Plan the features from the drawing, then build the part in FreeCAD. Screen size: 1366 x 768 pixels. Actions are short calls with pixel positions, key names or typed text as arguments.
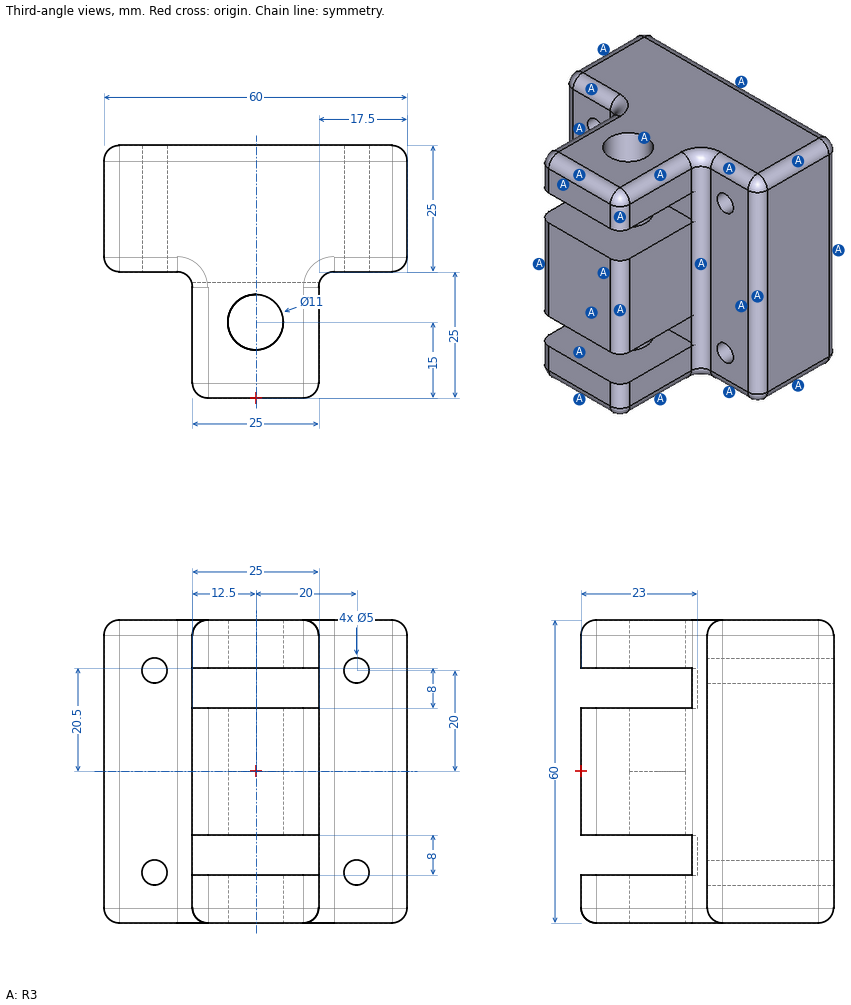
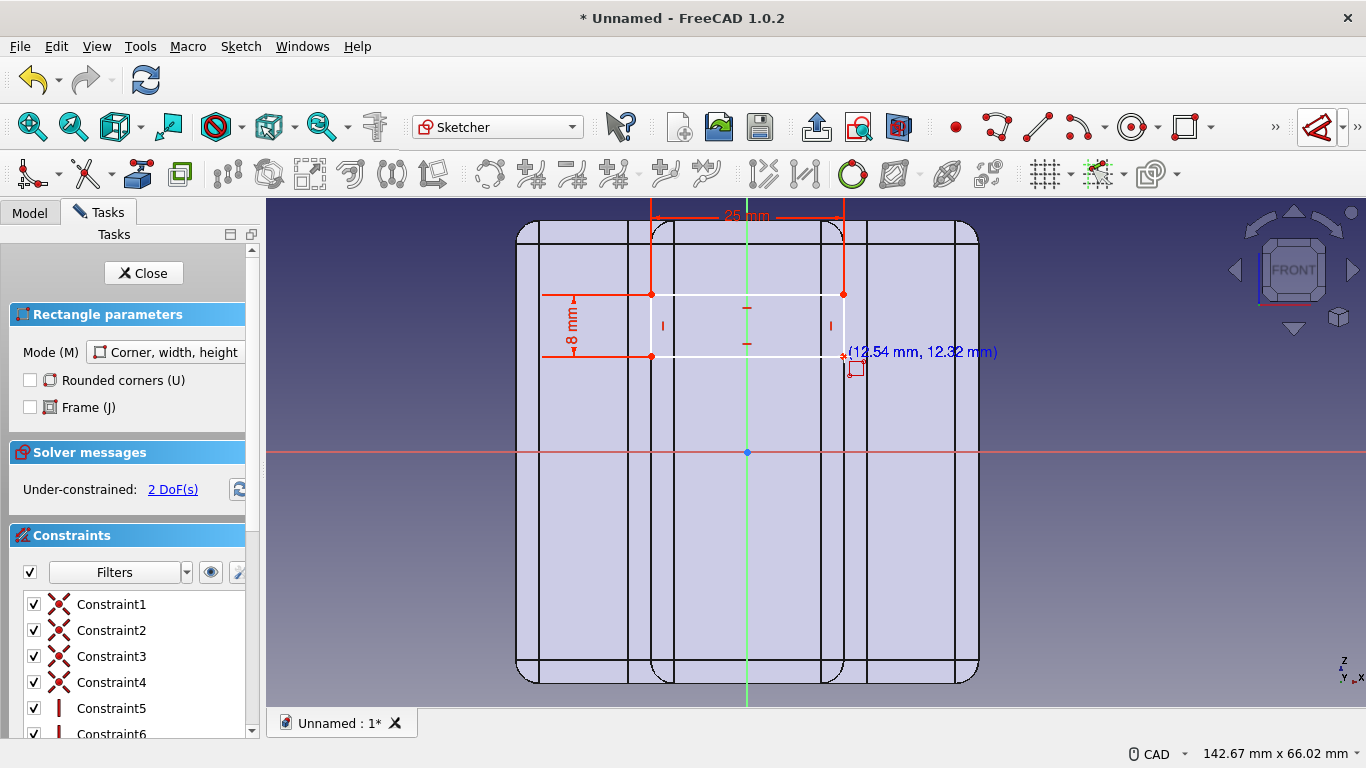
click(651, 548)
move(844, 610)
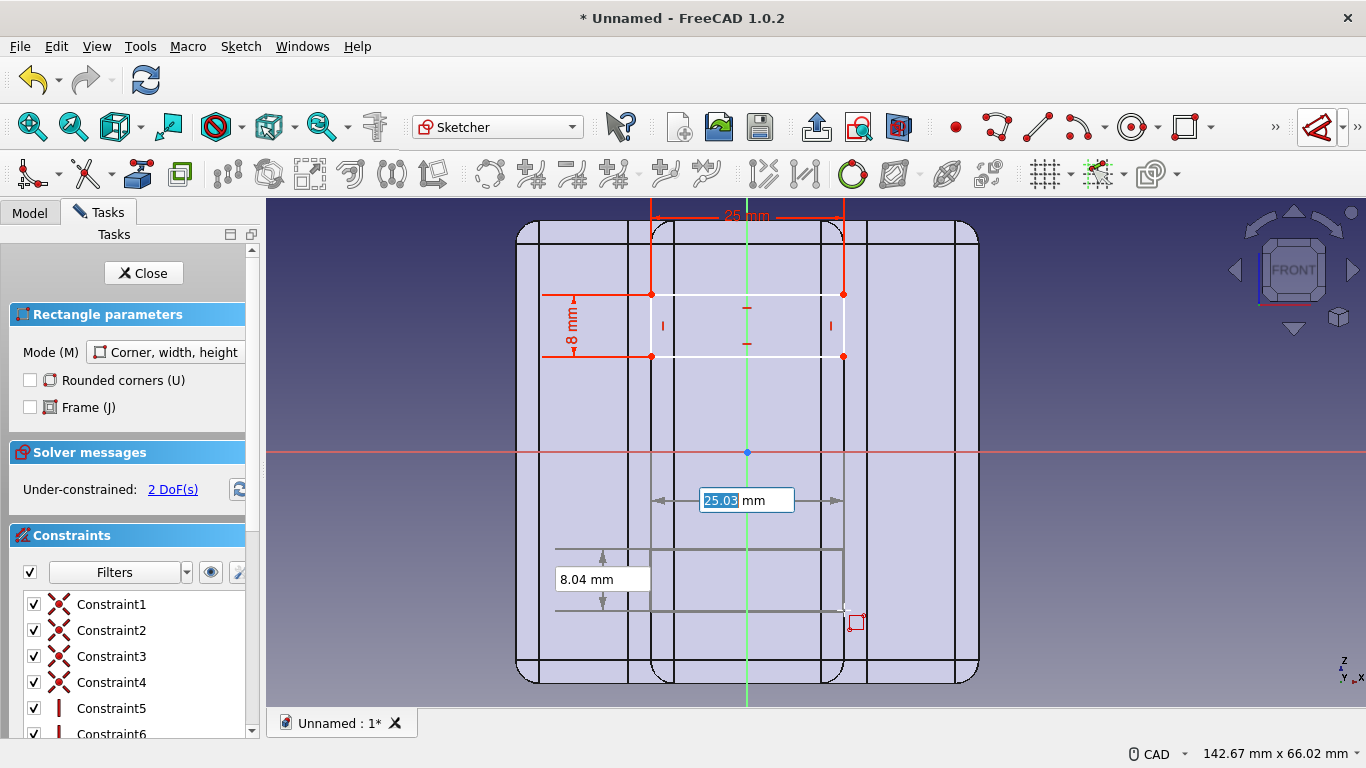
text(25)
key(Tab)
text(8)
key(Return)
key(Escape)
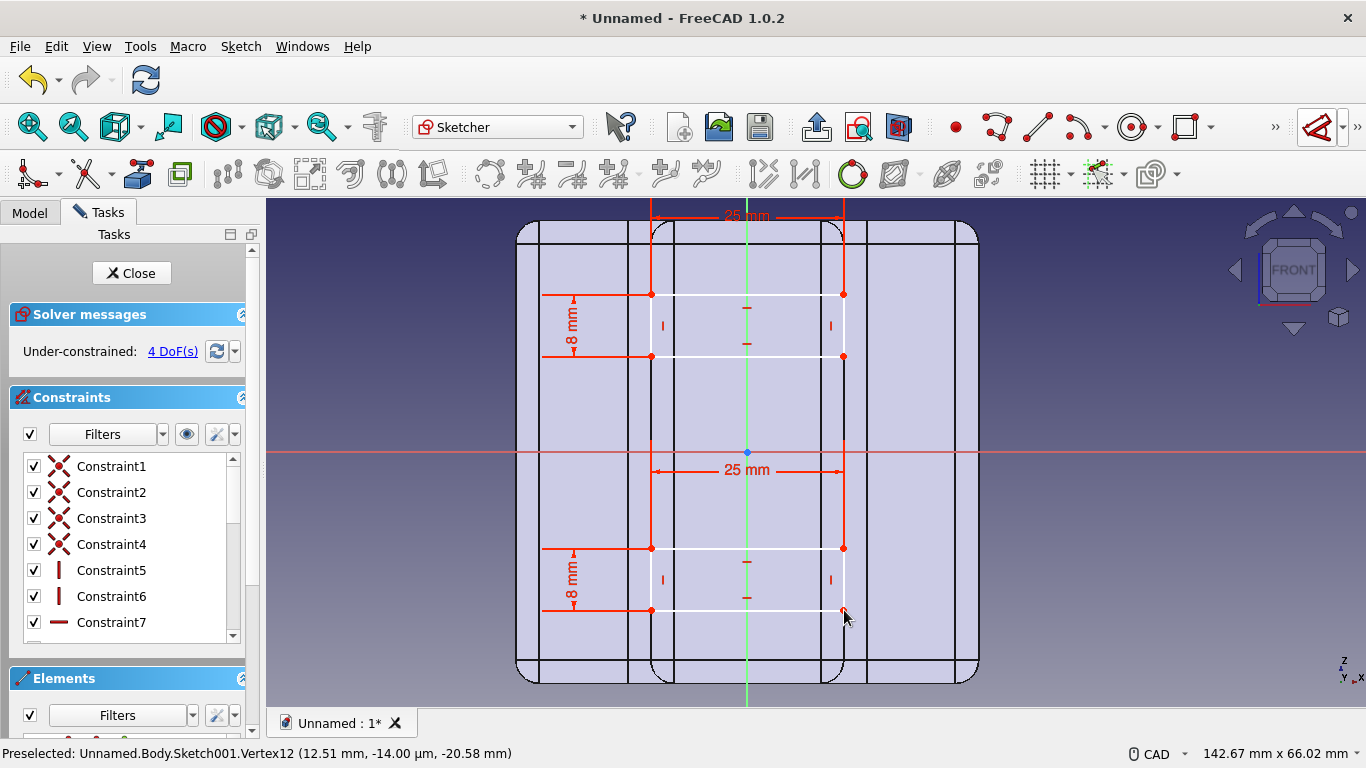
click(651, 357)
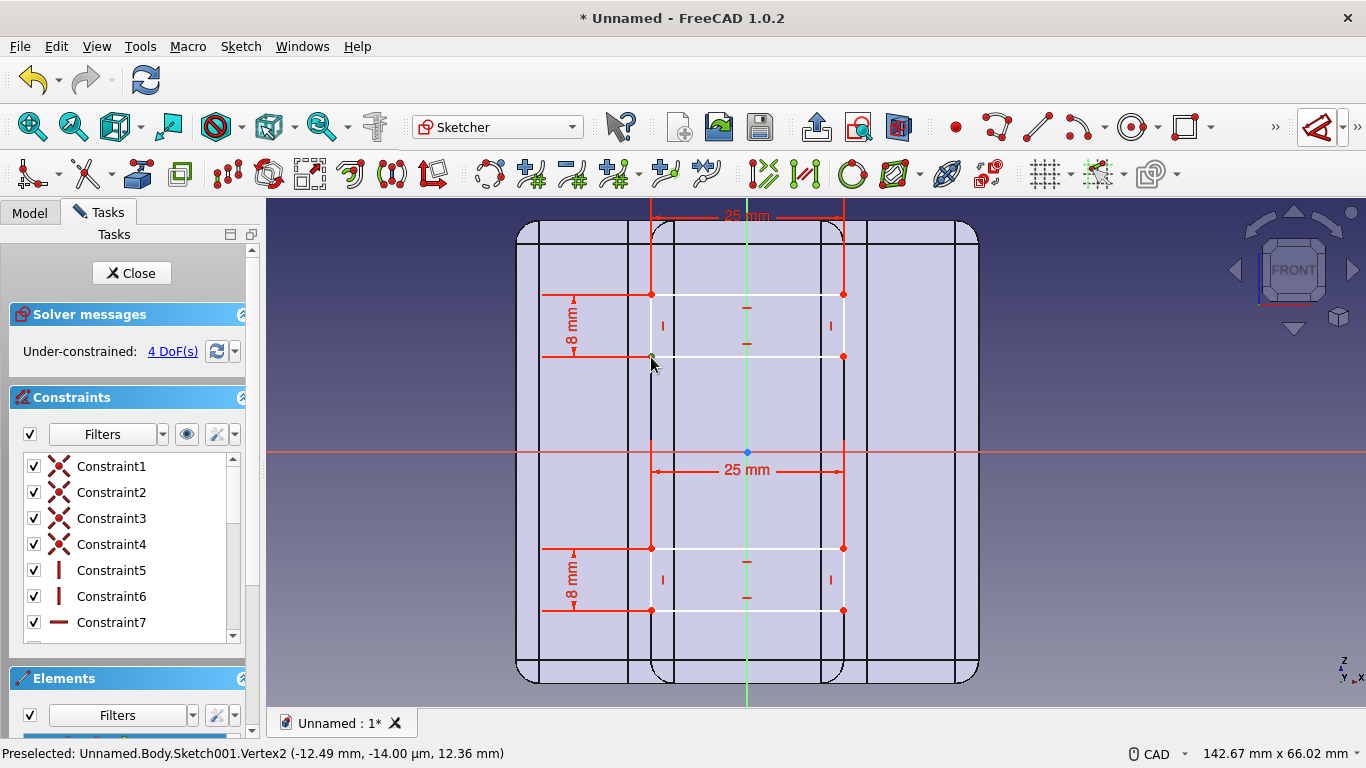
click(651, 549)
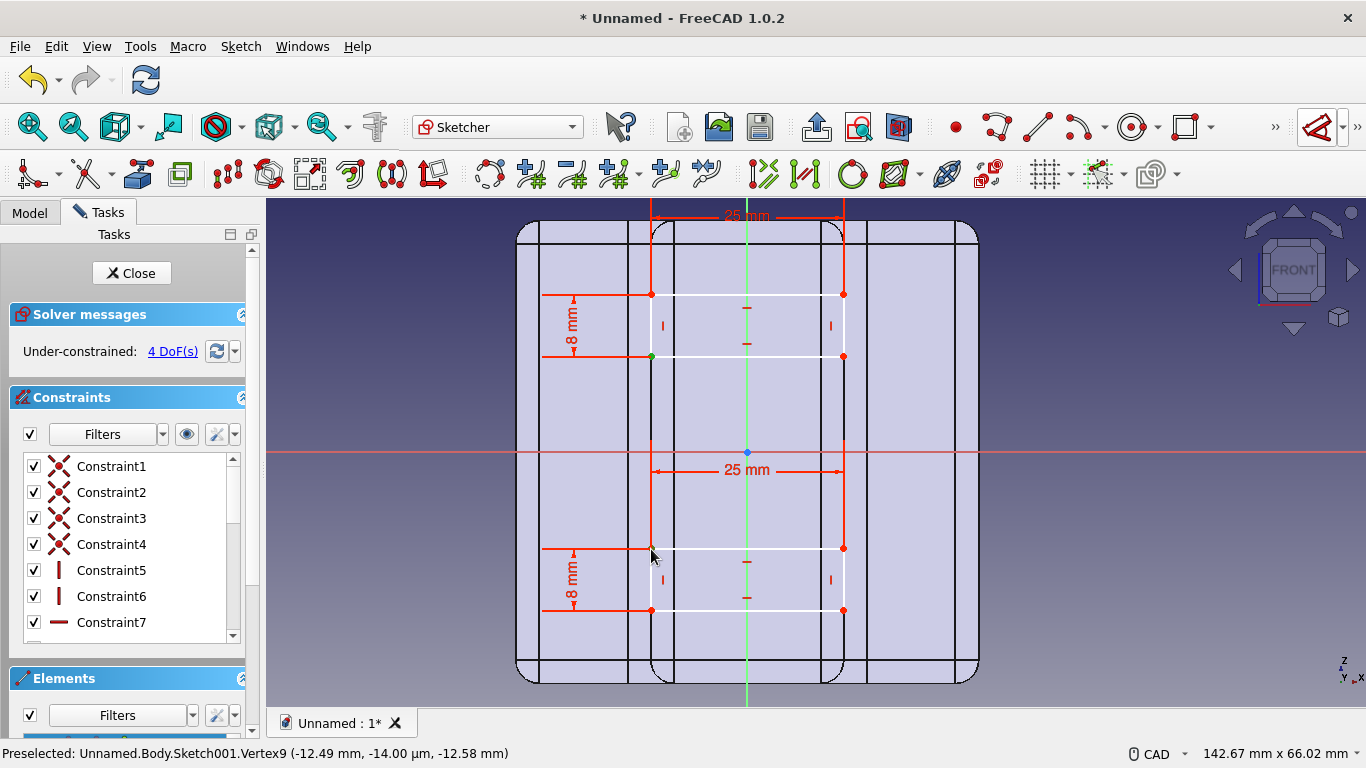
click(359, 452)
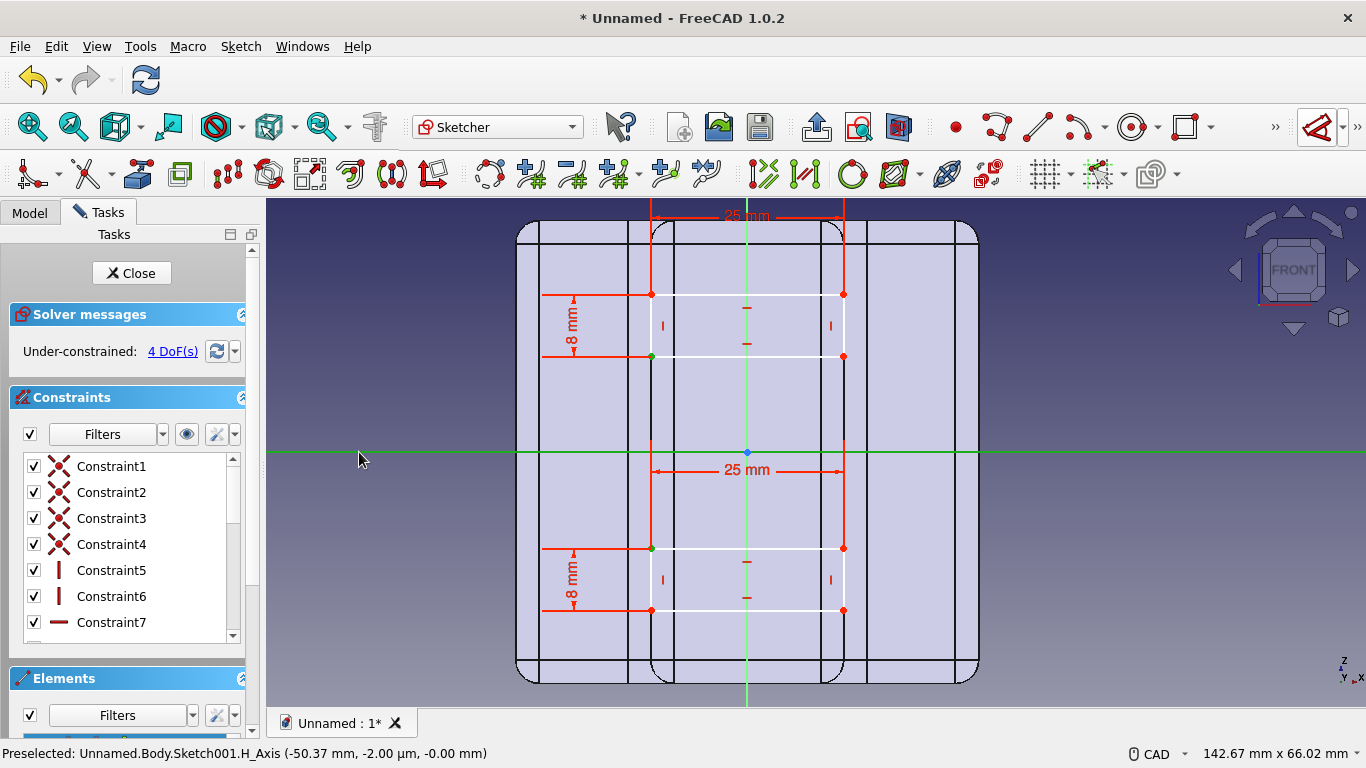
key(s)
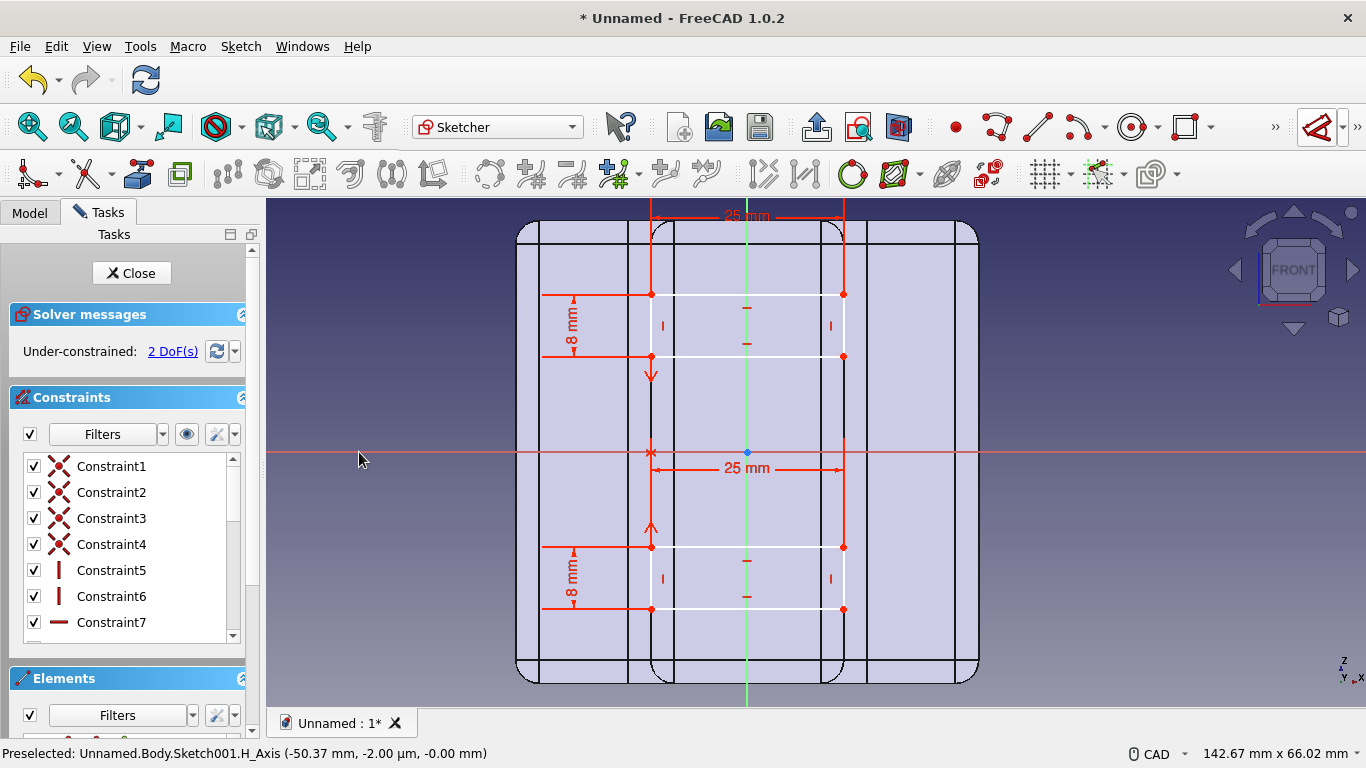
click(651, 295)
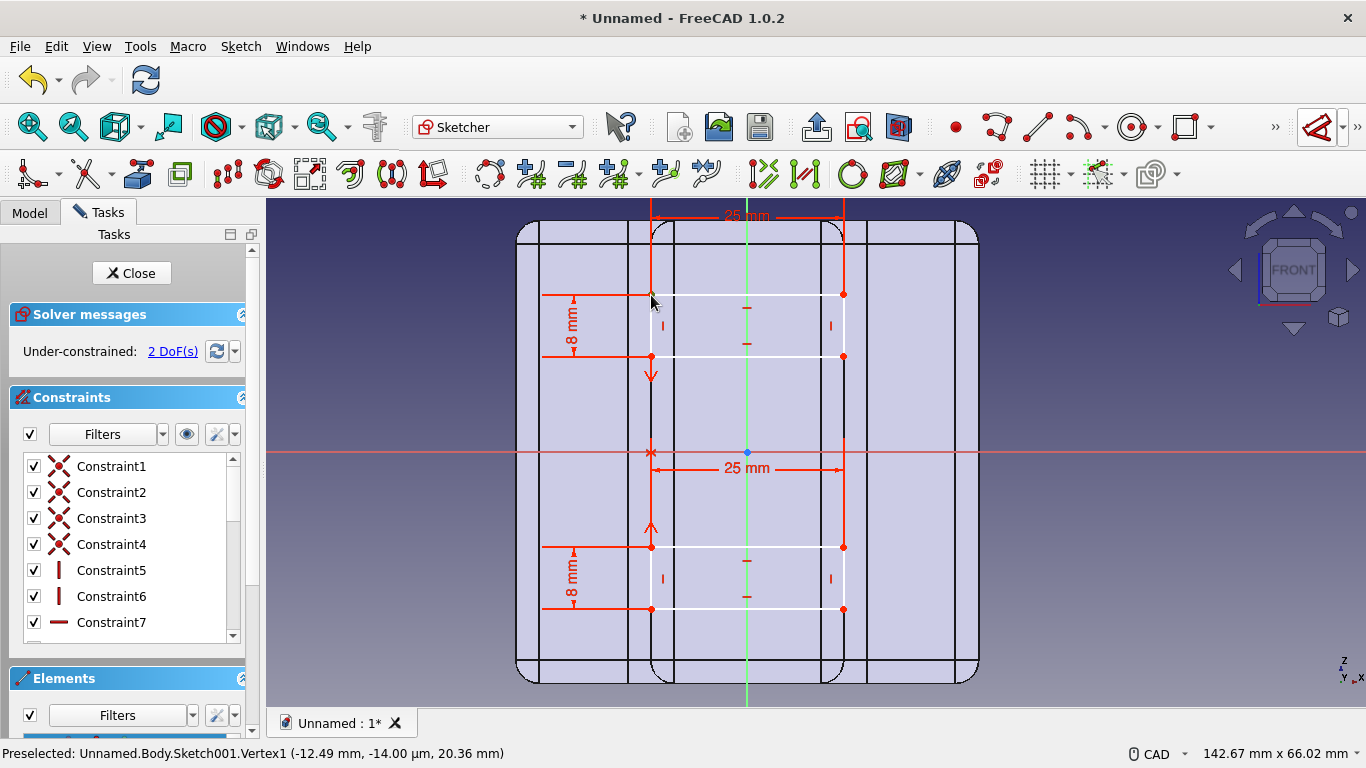
key(l)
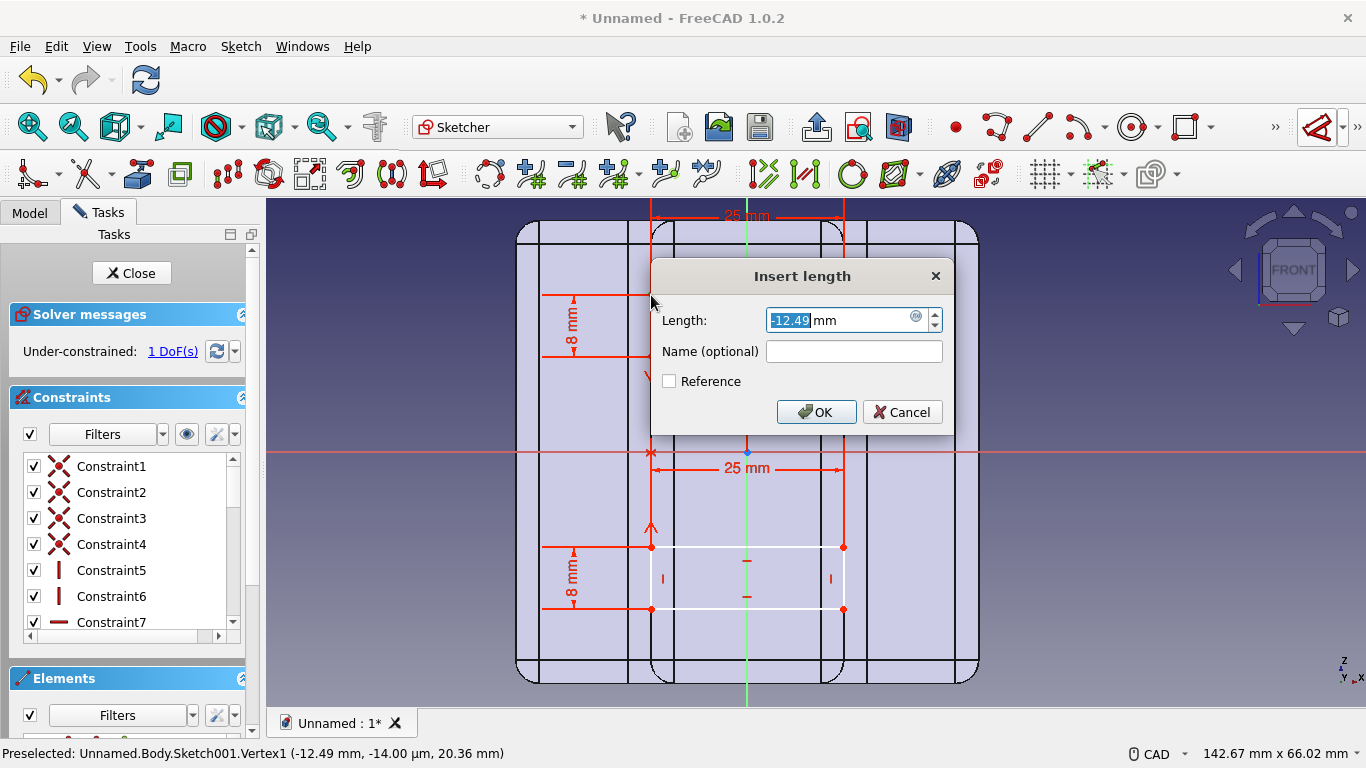
text(-12.5)
key(Return)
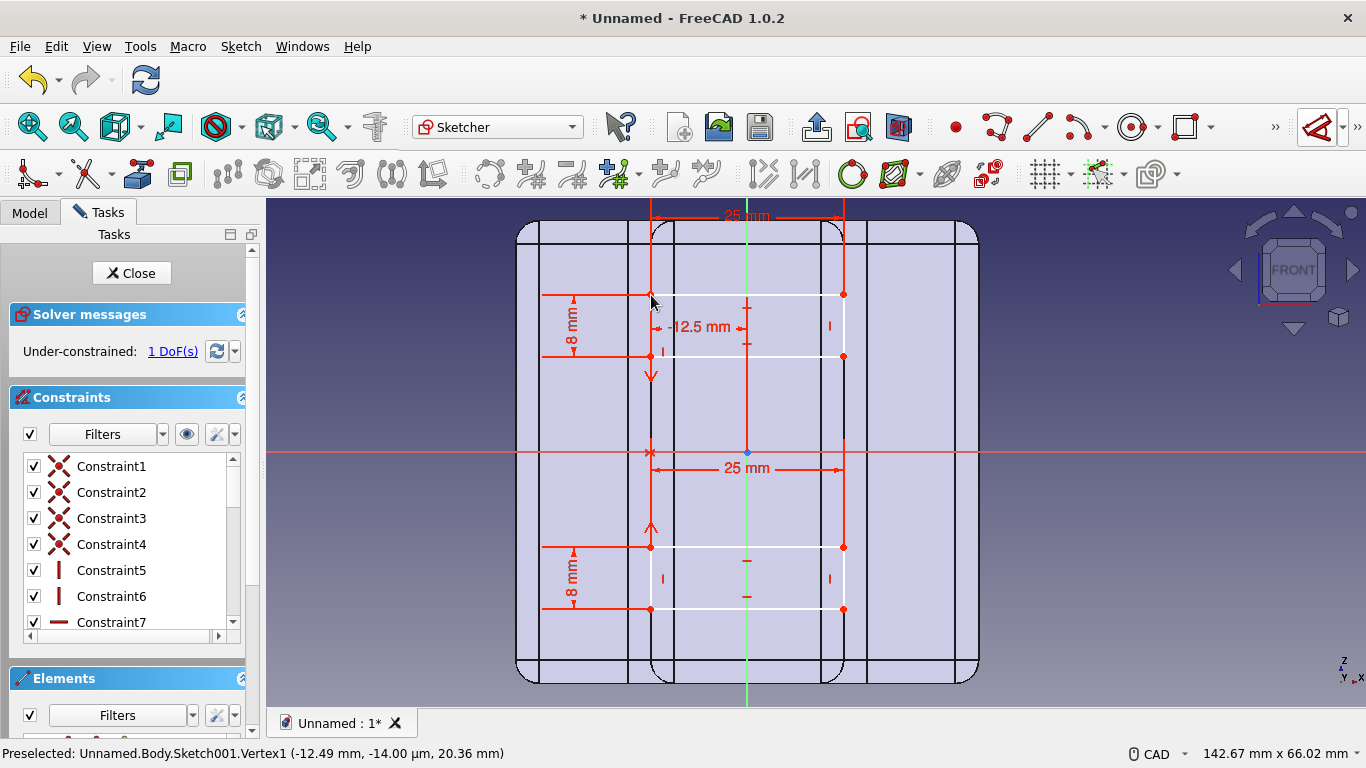
click(651, 295)